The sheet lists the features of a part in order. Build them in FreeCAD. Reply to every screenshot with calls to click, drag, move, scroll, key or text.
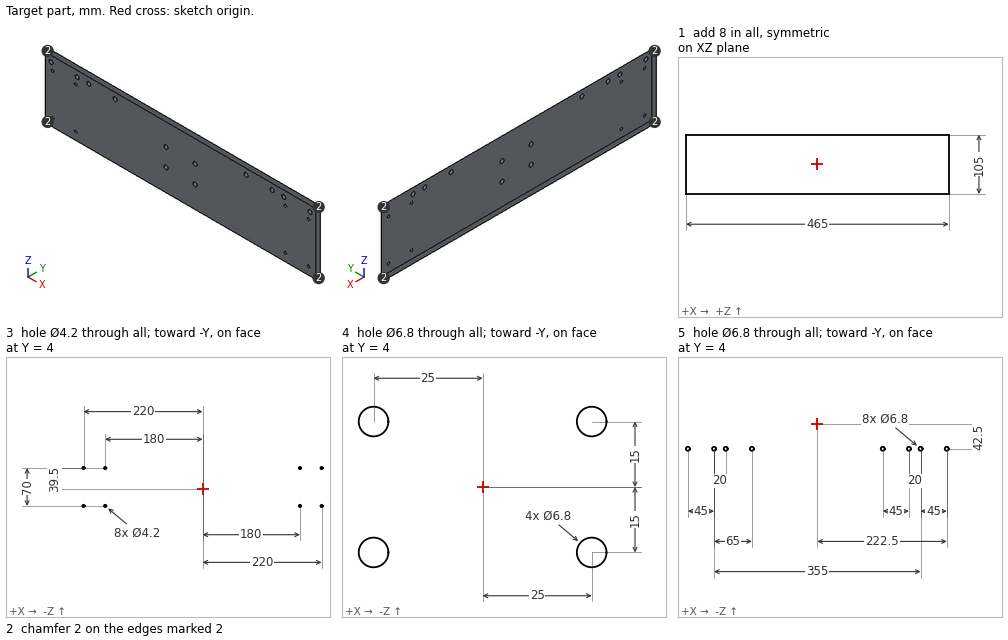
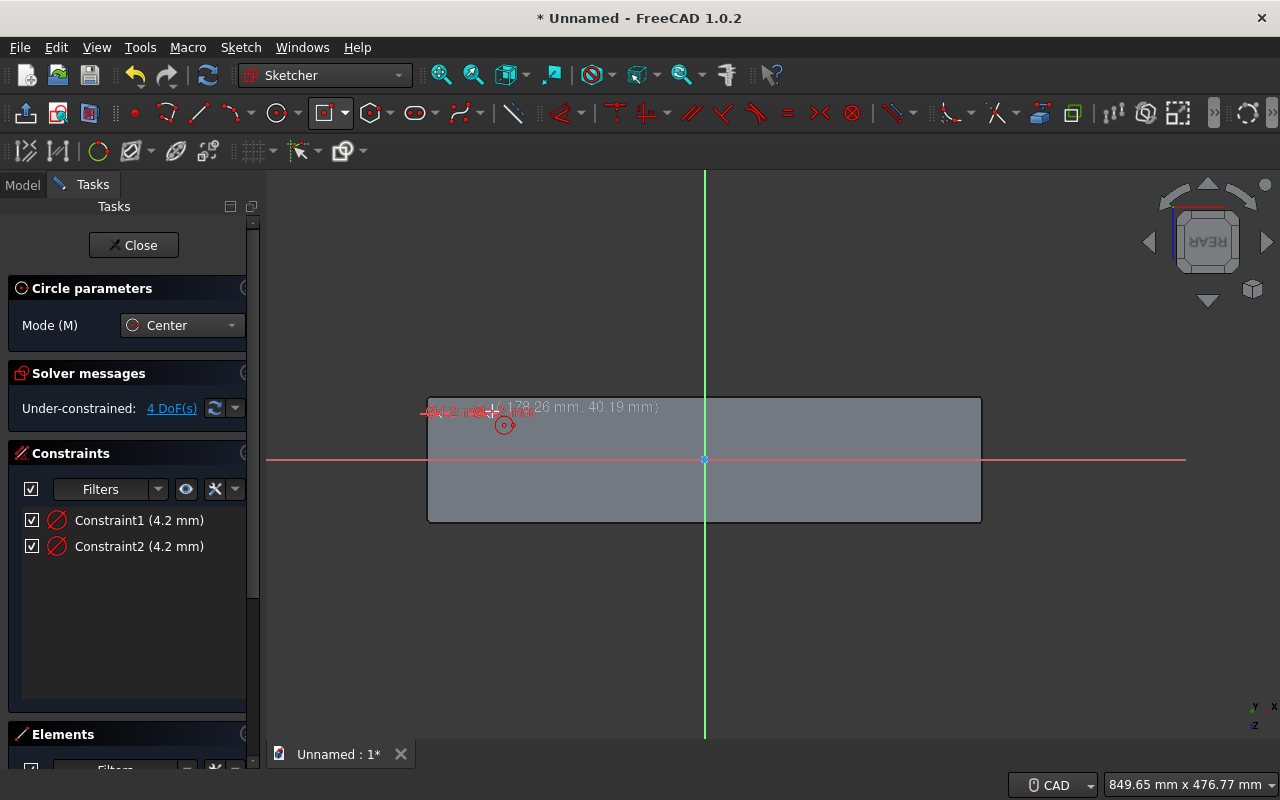
scroll(490, 496, up, 12)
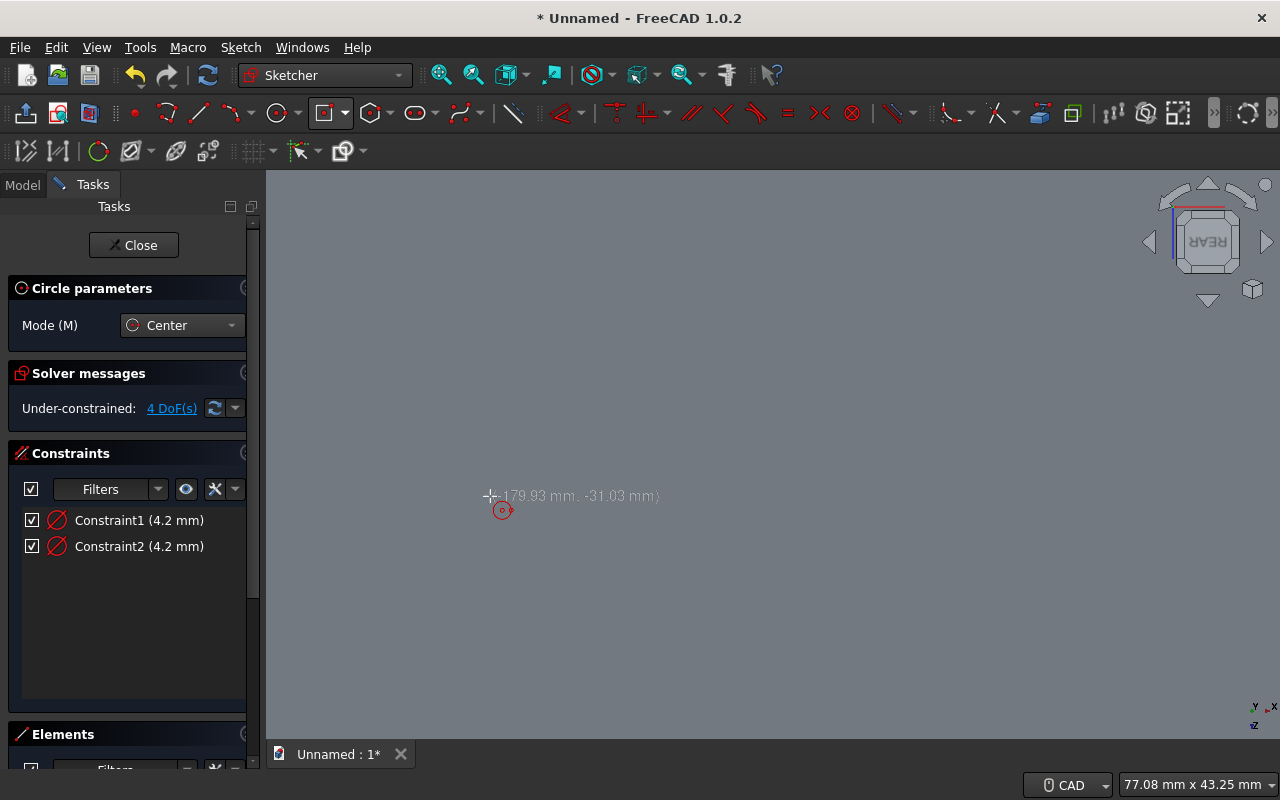
scroll(490, 496, down, 12)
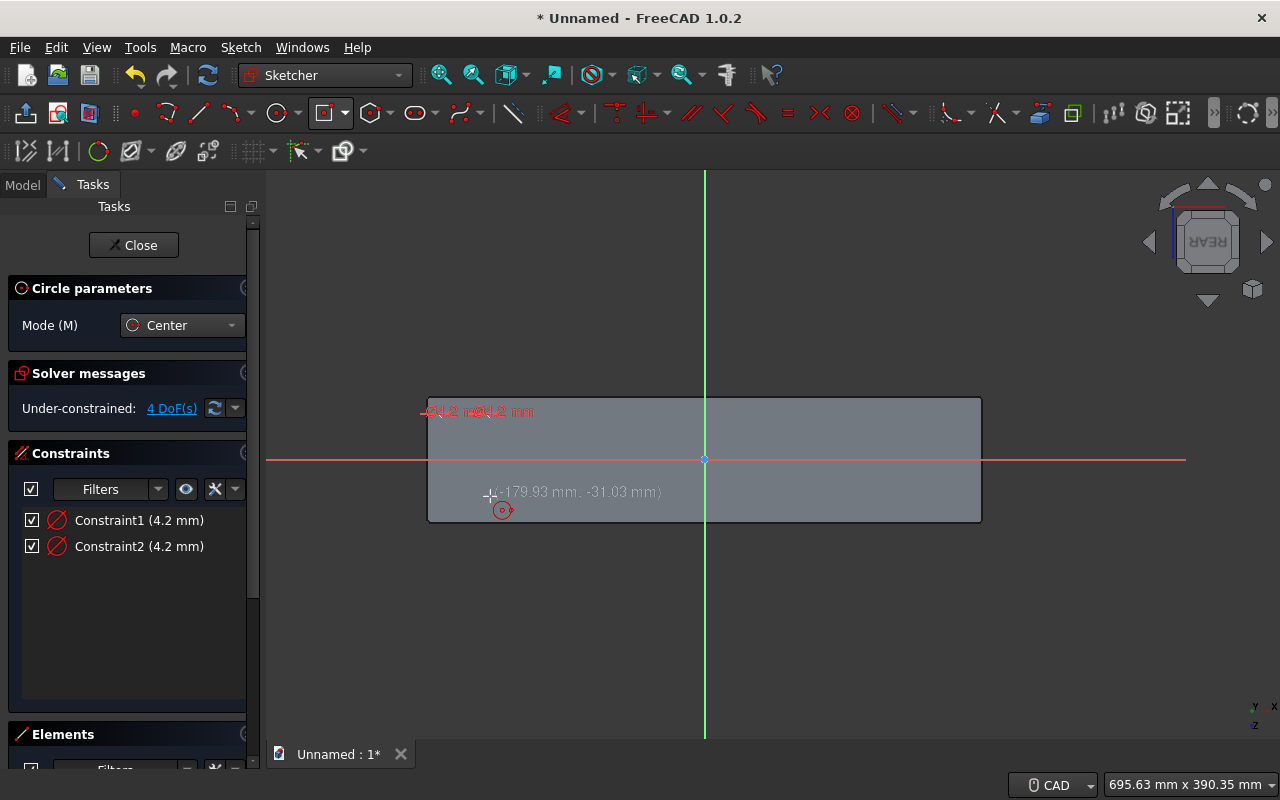
click(490, 496)
move(492, 495)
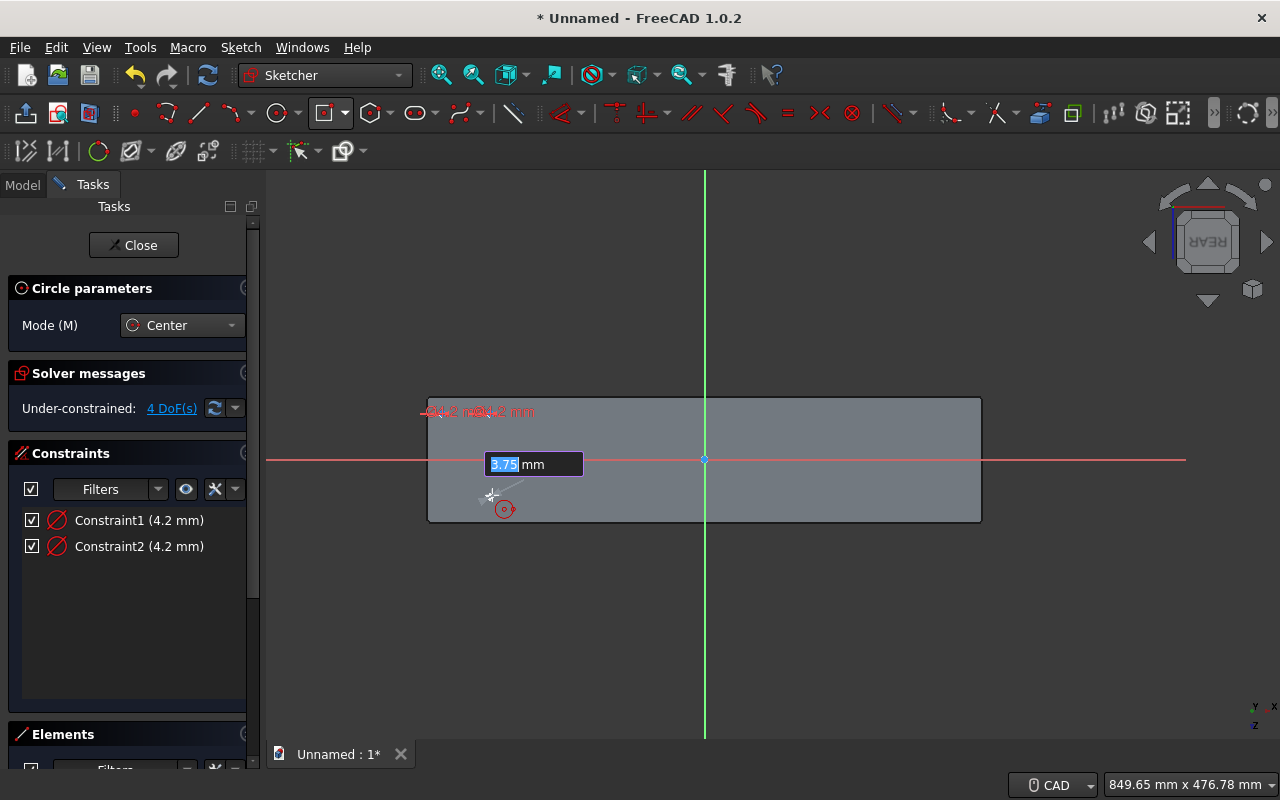
text(4.2)
key(Return)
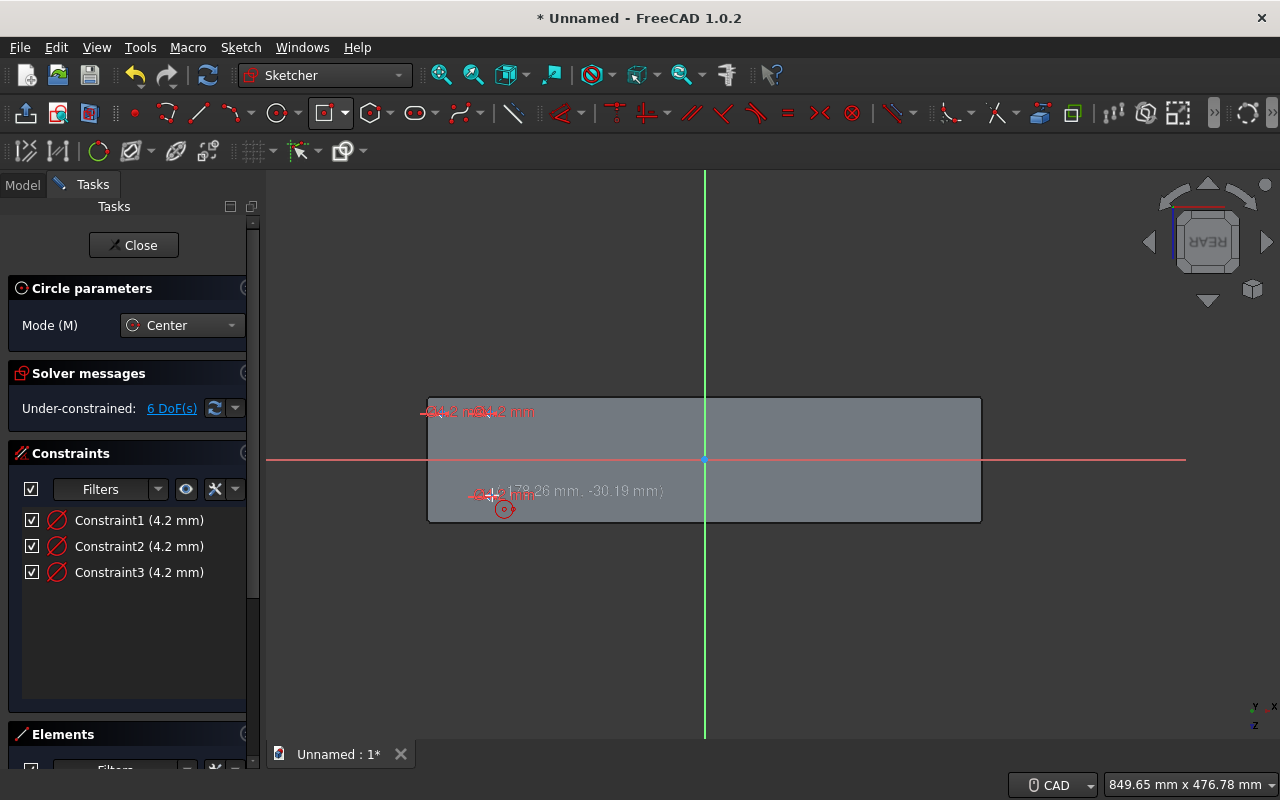
scroll(442, 496, up, 12)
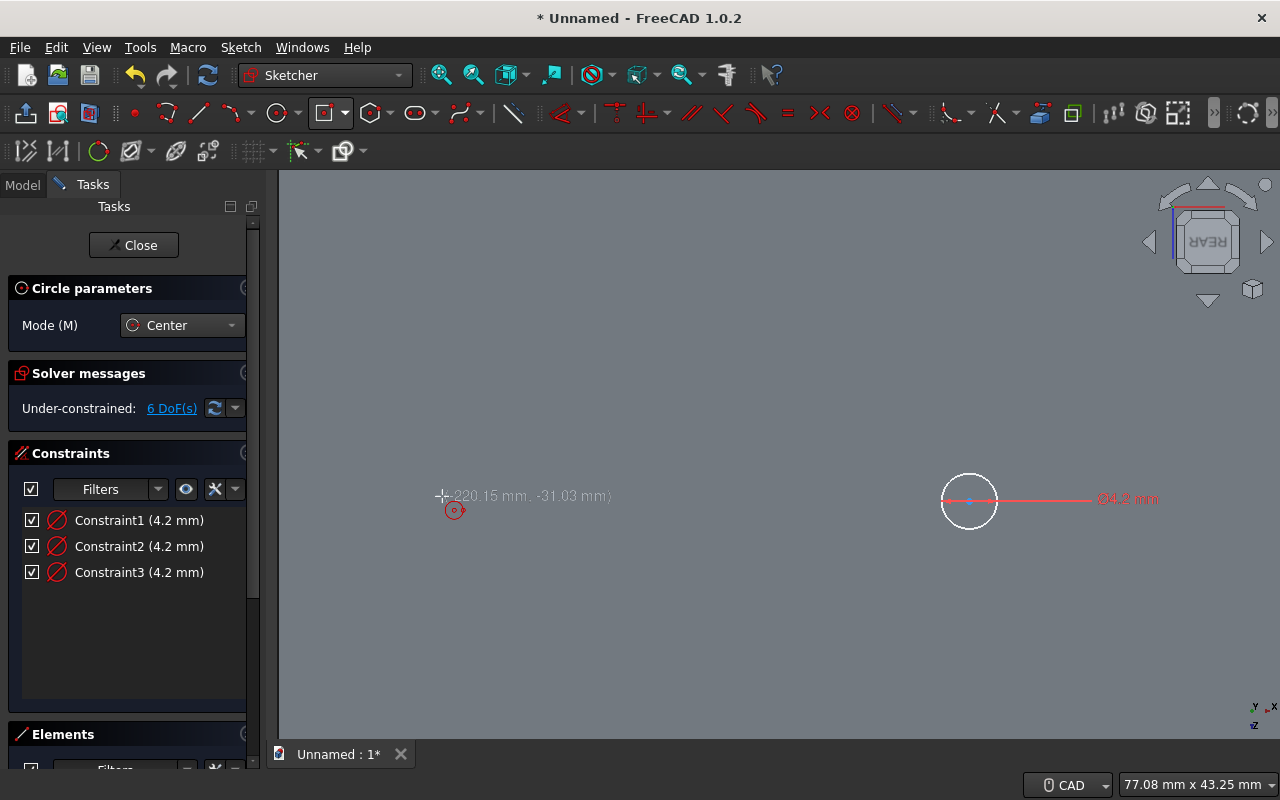
scroll(442, 496, down, 12)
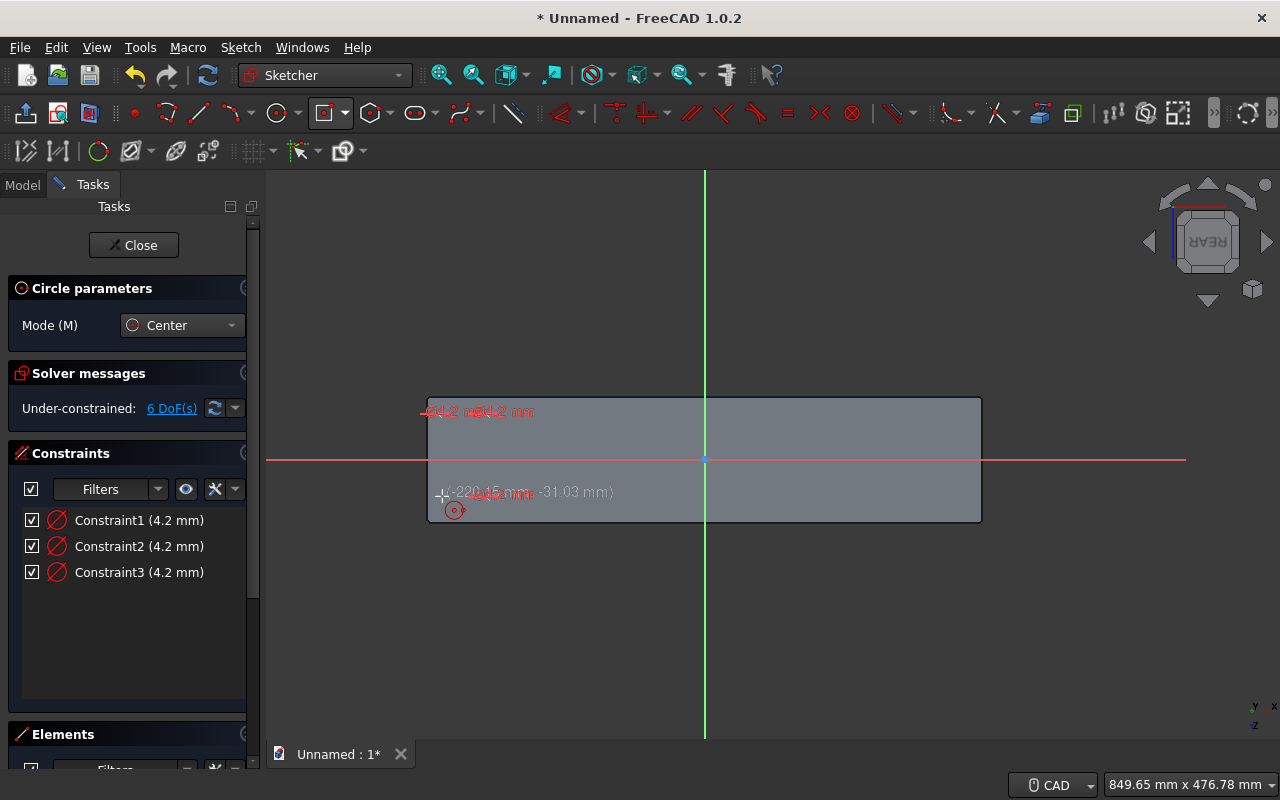
click(442, 496)
move(444, 495)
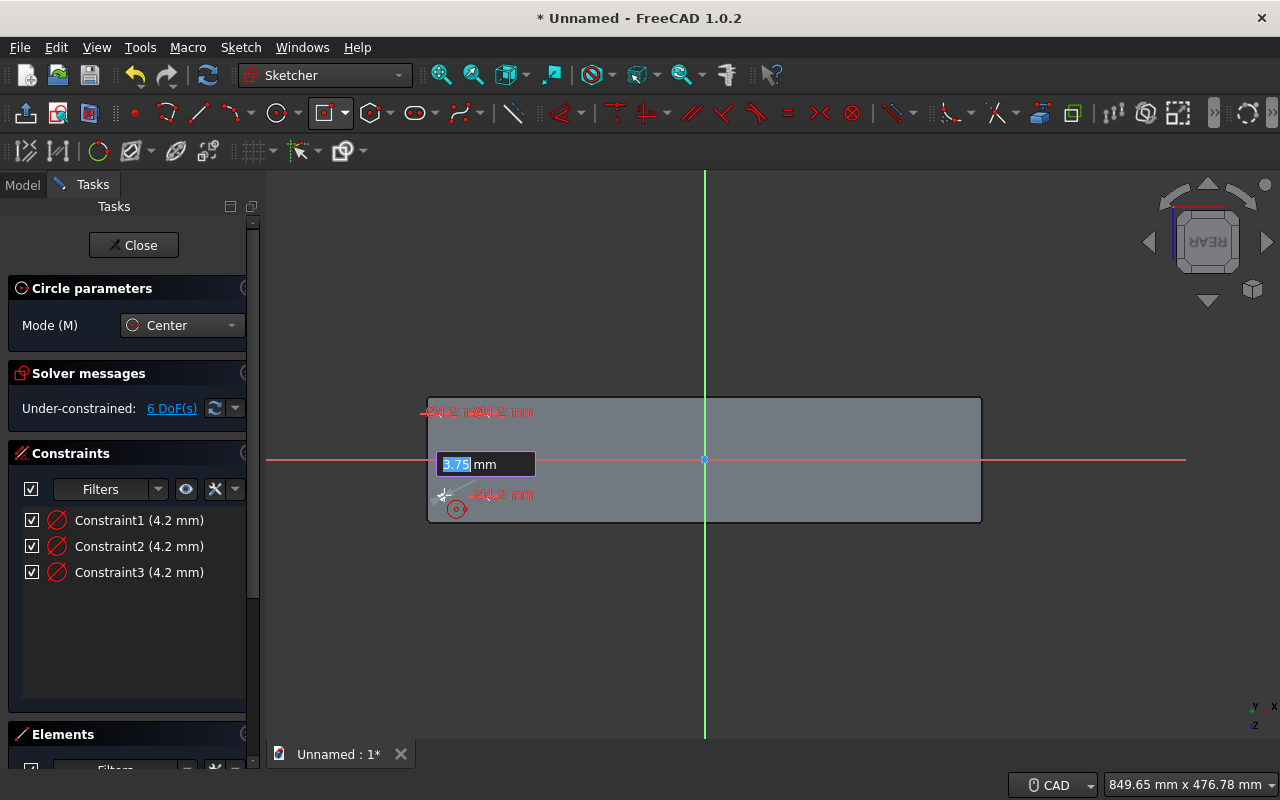
text(4.2)
key(Return)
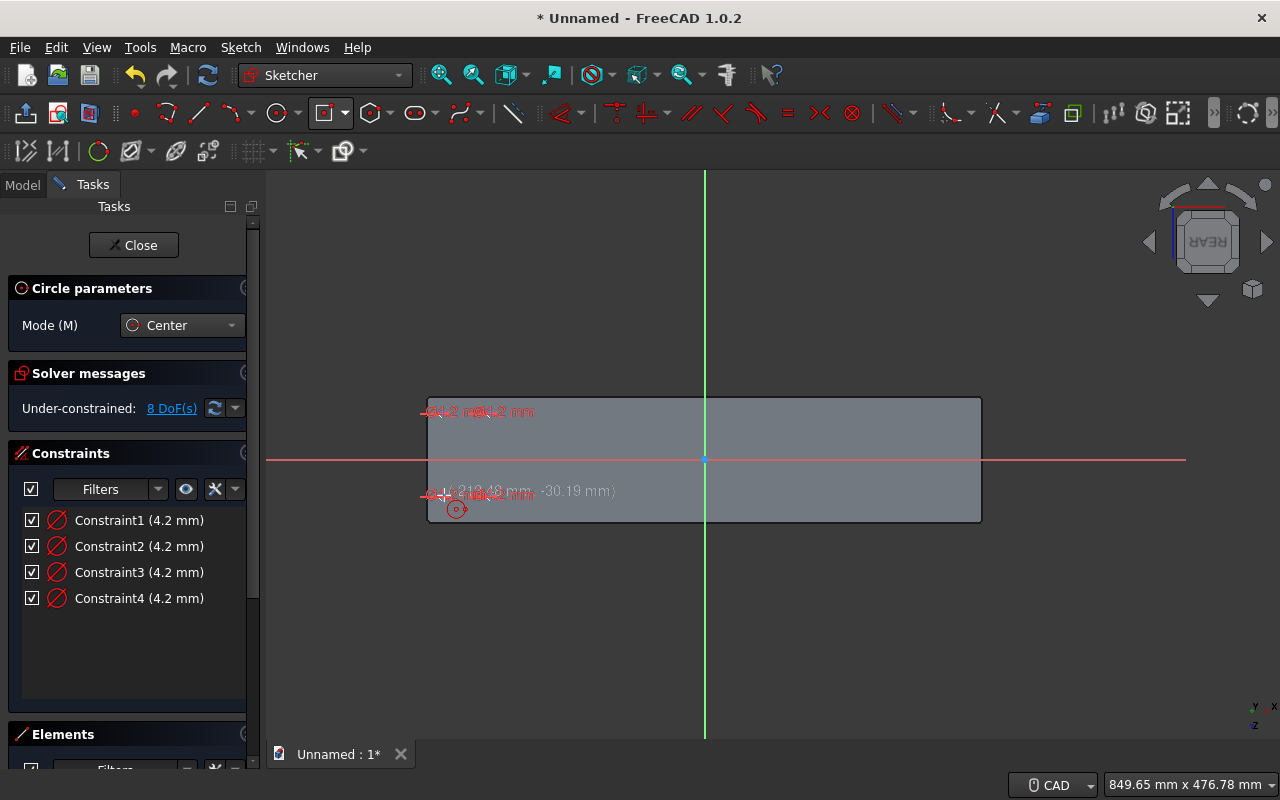
scroll(967, 496, up, 12)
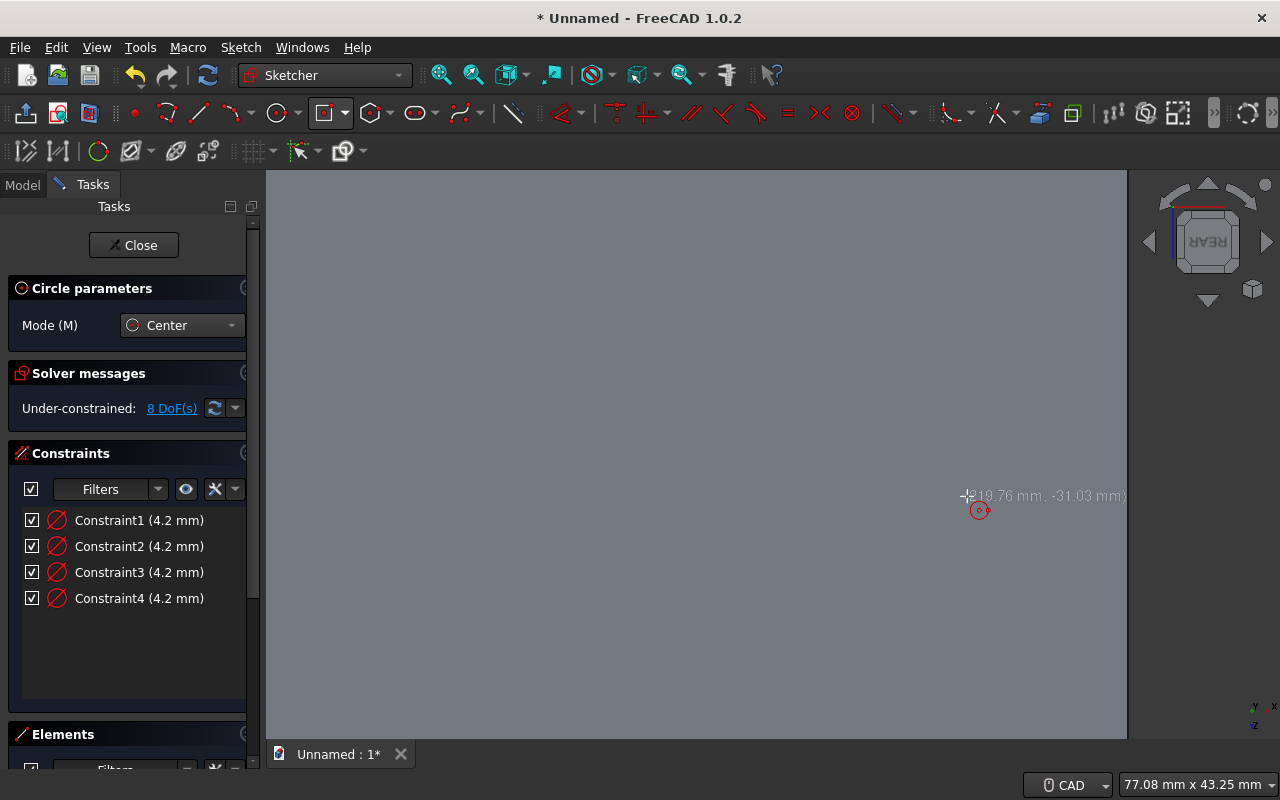
scroll(967, 496, down, 12)